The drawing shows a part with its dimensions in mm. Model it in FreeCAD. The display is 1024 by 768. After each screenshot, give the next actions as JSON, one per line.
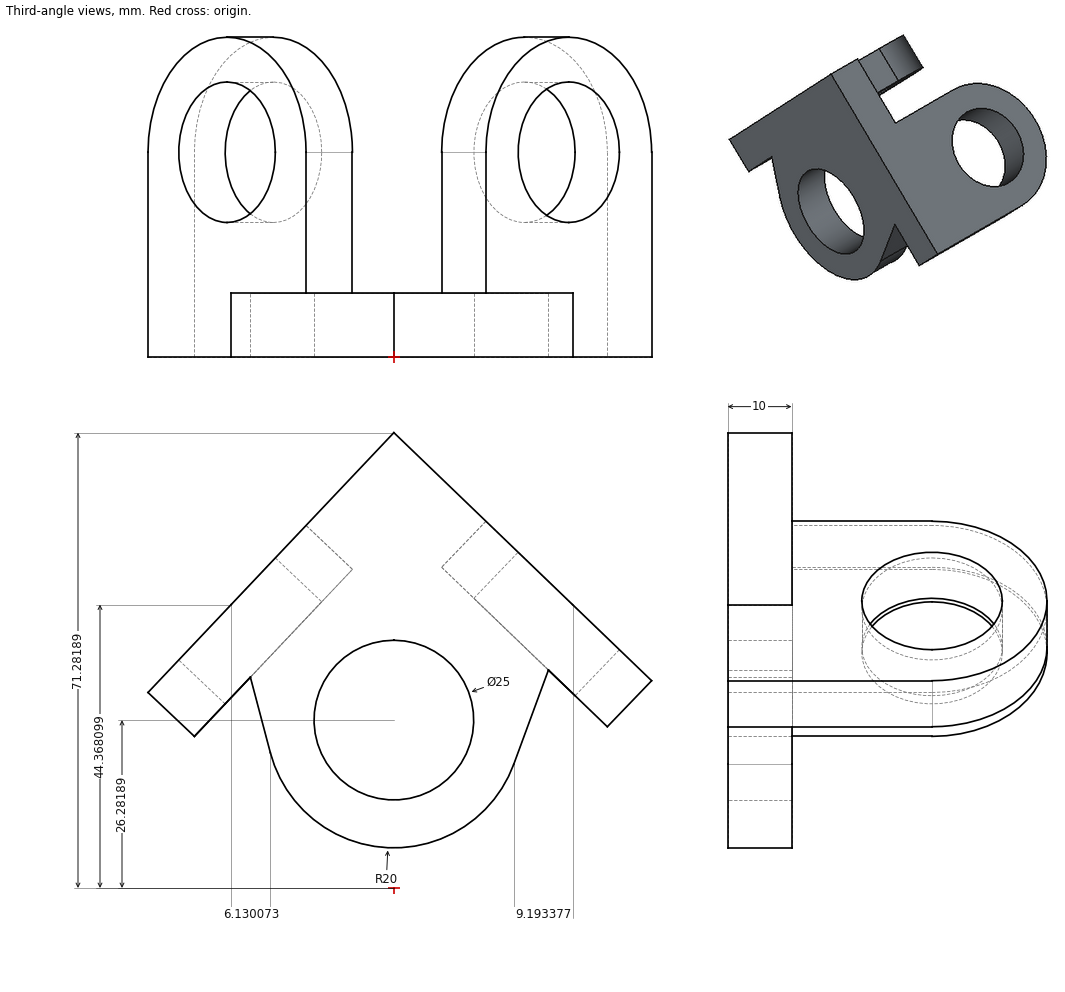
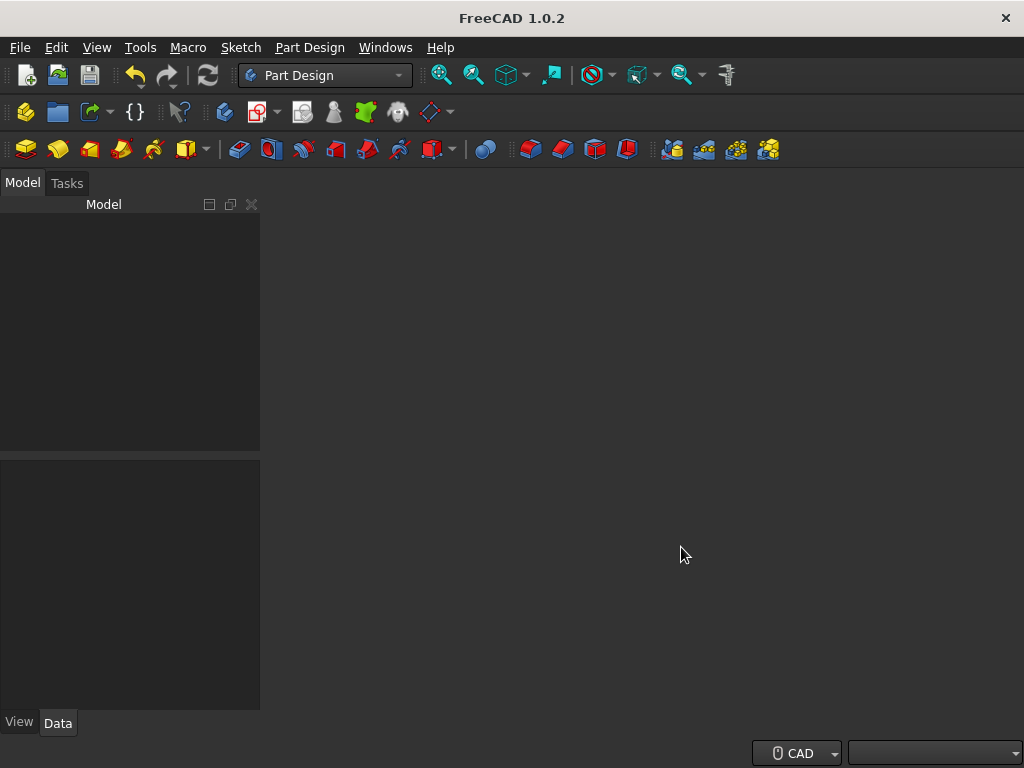
{"action": "left_click", "coordinate": [26, 76]}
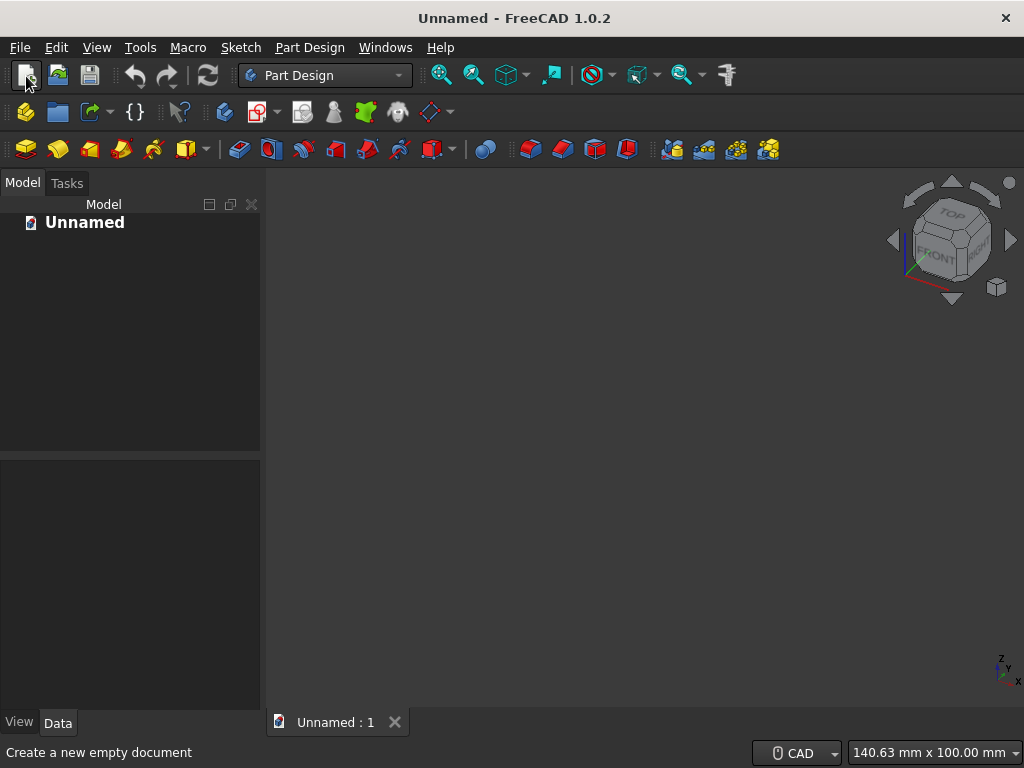
{"action": "left_click", "coordinate": [258, 112]}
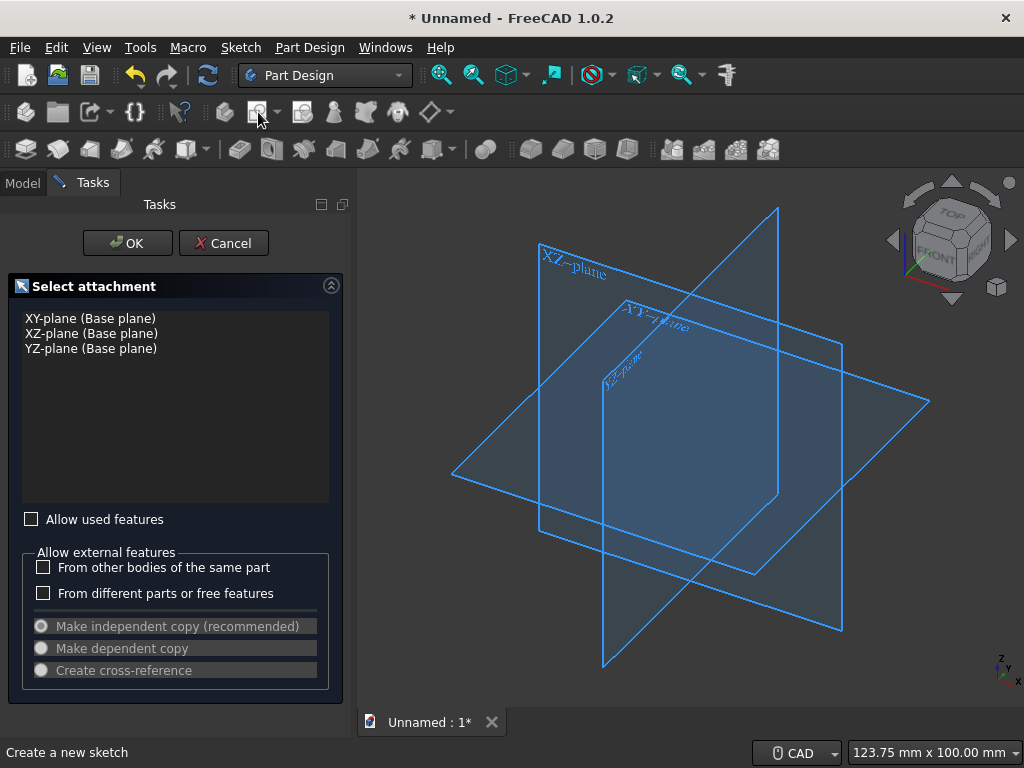
{"action": "left_click", "coordinate": [82, 334]}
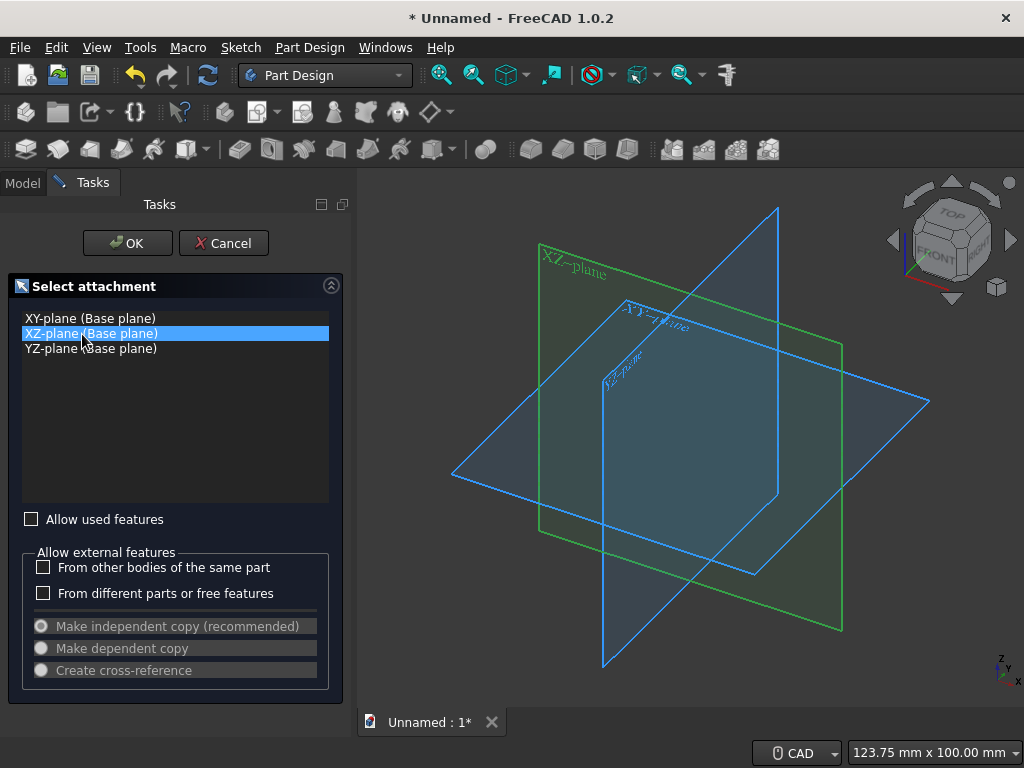
{"action": "left_click", "coordinate": [128, 243]}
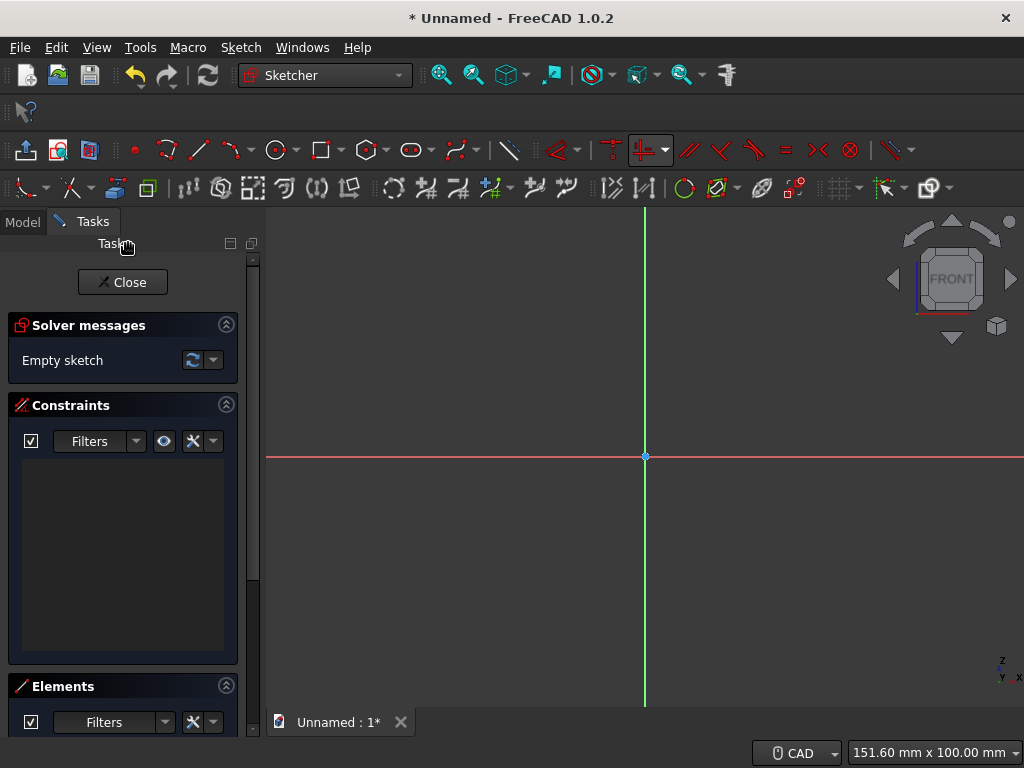
{"action": "scroll", "coordinate": [425, 679], "scroll_direction": "down", "scroll_amount": 2}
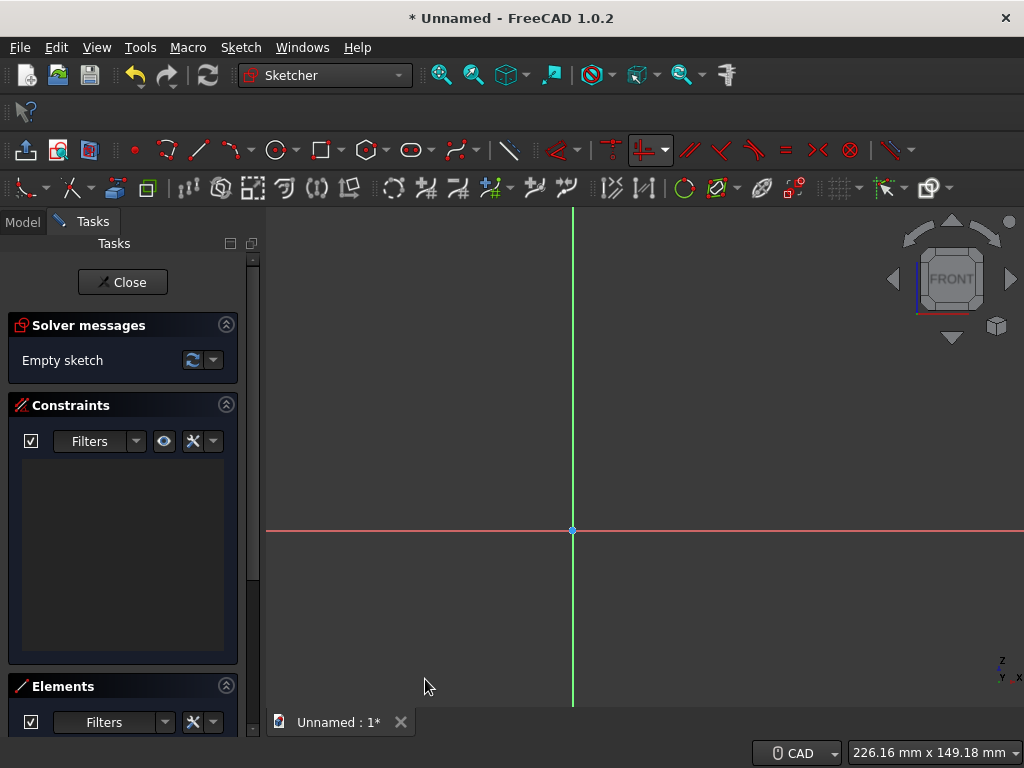
{"action": "left_click", "coordinate": [168, 150]}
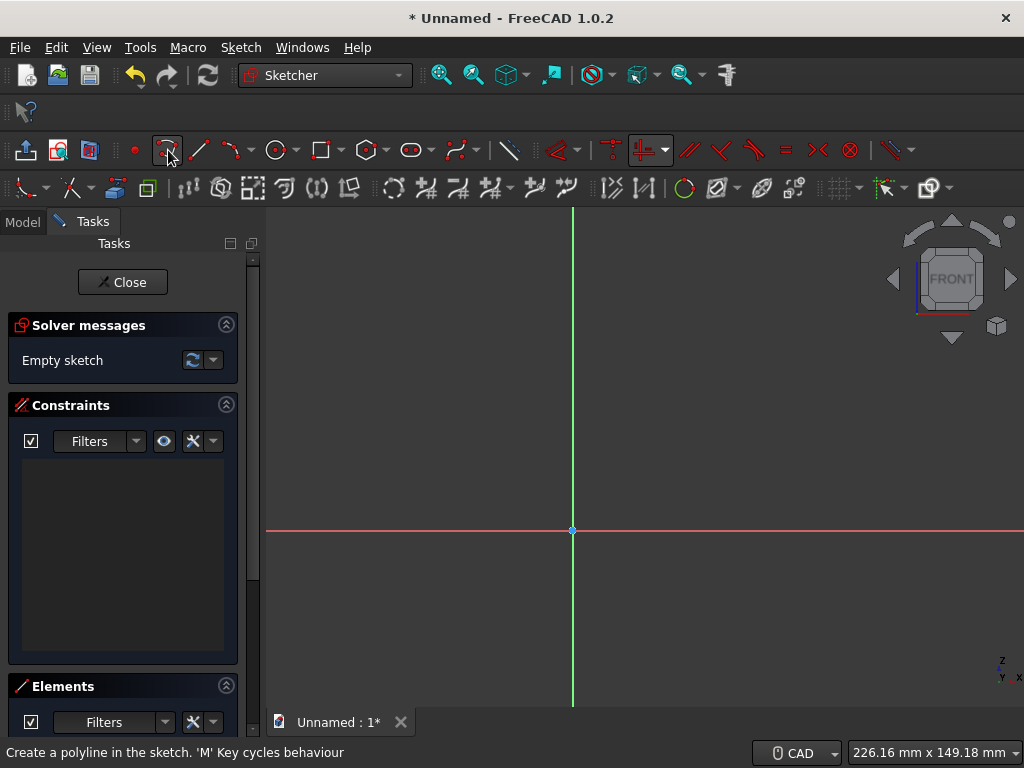
{"action": "left_click", "coordinate": [508, 460]}
{"action": "left_click", "coordinate": [487, 382]}
{"action": "left_click", "coordinate": [573, 292]}
{"action": "left_click", "coordinate": [666, 382]}
{"action": "left_click", "coordinate": [635, 466]}
{"action": "right_click", "coordinate": [635, 466]}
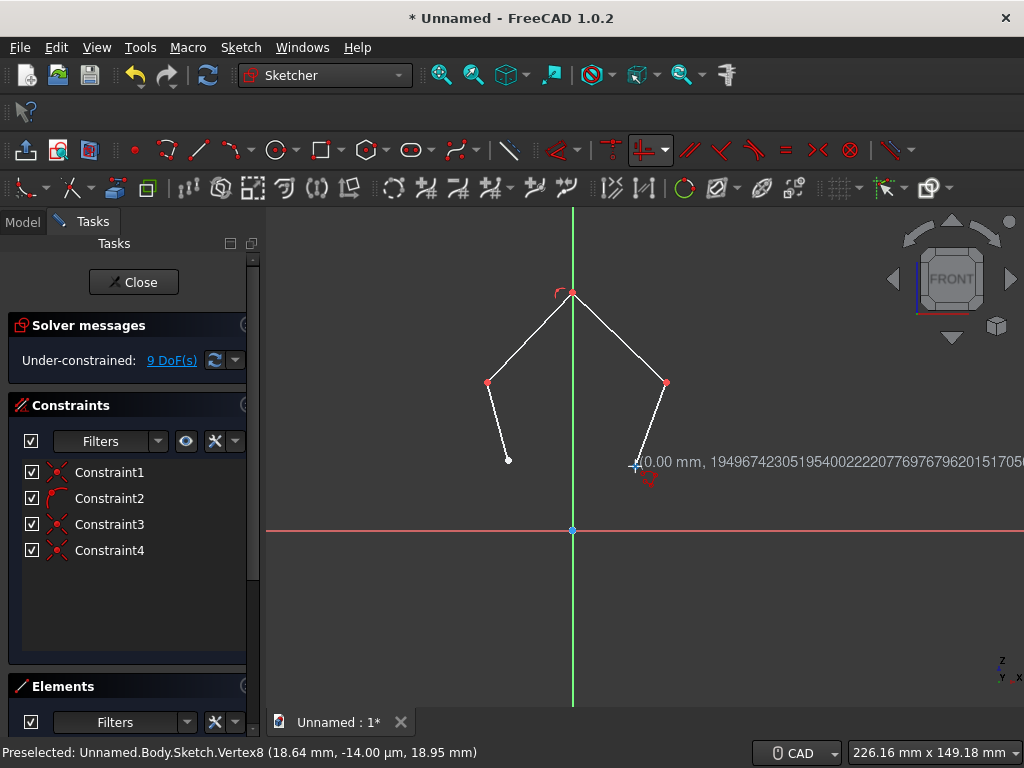
{"action": "left_click", "coordinate": [232, 150]}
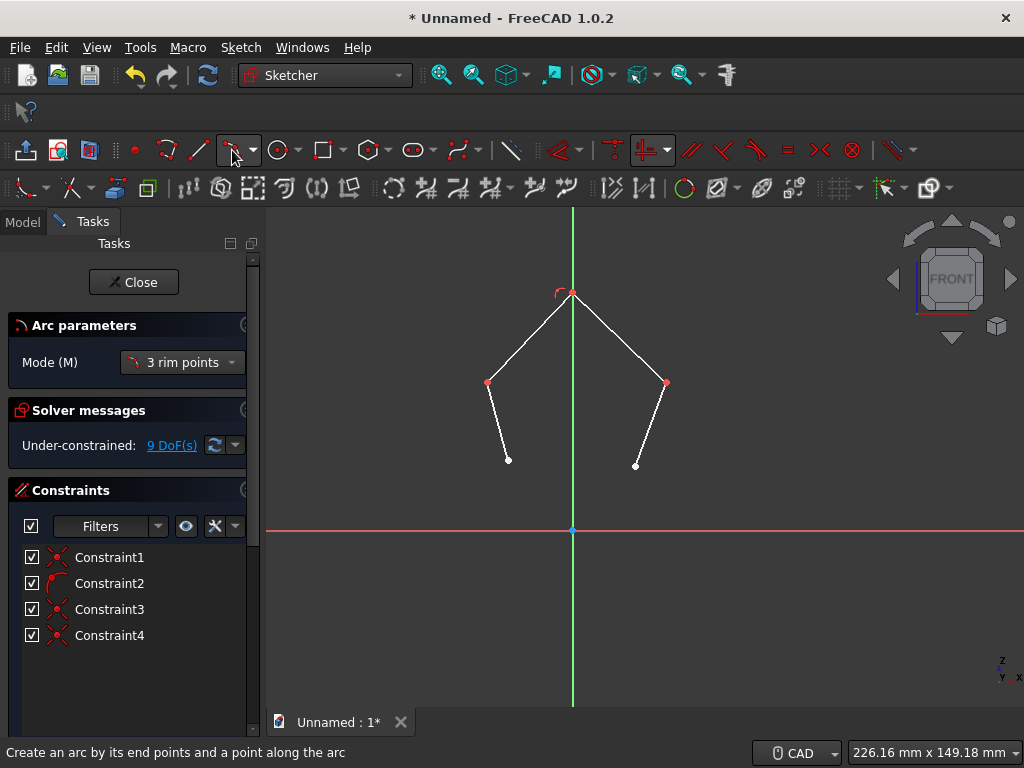
{"action": "left_click", "coordinate": [635, 467]}
{"action": "left_click", "coordinate": [508, 461]}
{"action": "left_click", "coordinate": [553, 506]}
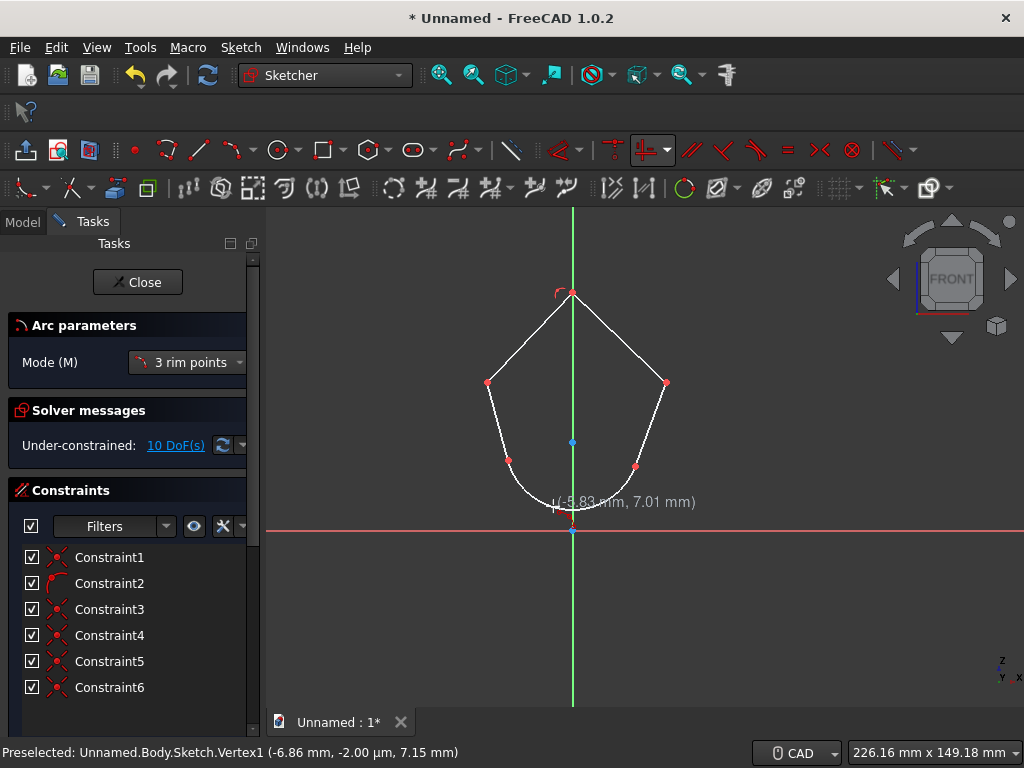
{"action": "left_click", "coordinate": [278, 150]}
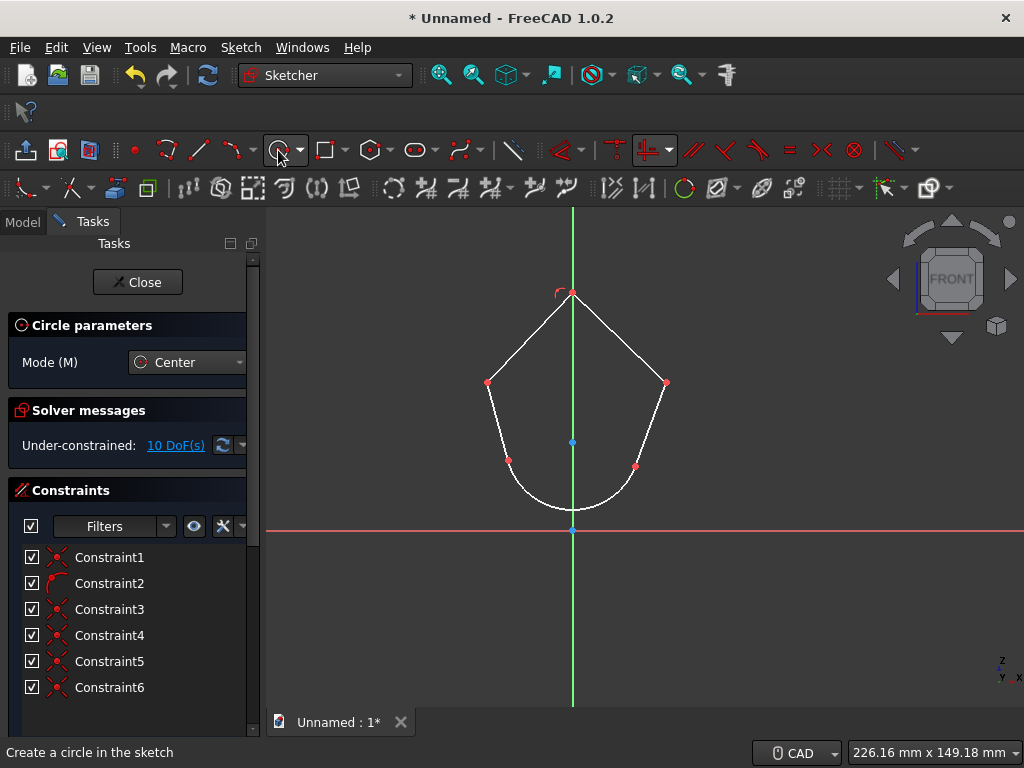
{"action": "left_click", "coordinate": [573, 442]}
{"action": "mouse_move", "coordinate": [602, 413]}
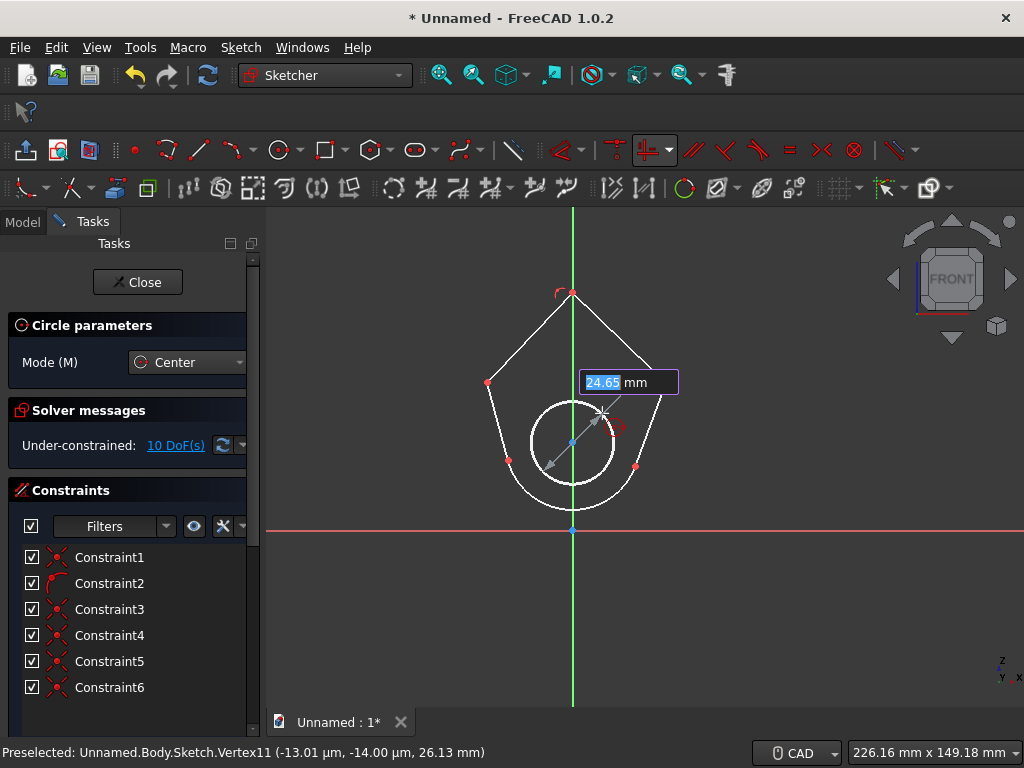
{"action": "type", "text": "25"}
{"action": "key", "text": "Return"}
{"action": "key", "text": "Escape"}